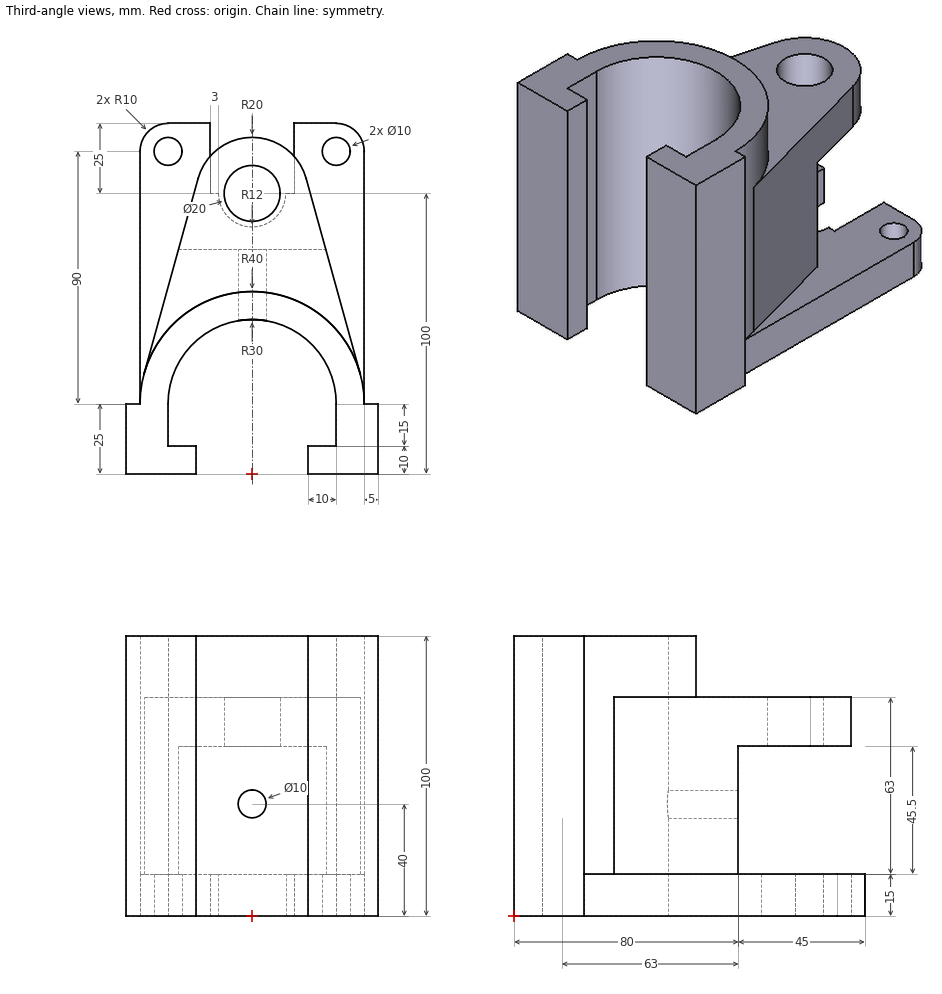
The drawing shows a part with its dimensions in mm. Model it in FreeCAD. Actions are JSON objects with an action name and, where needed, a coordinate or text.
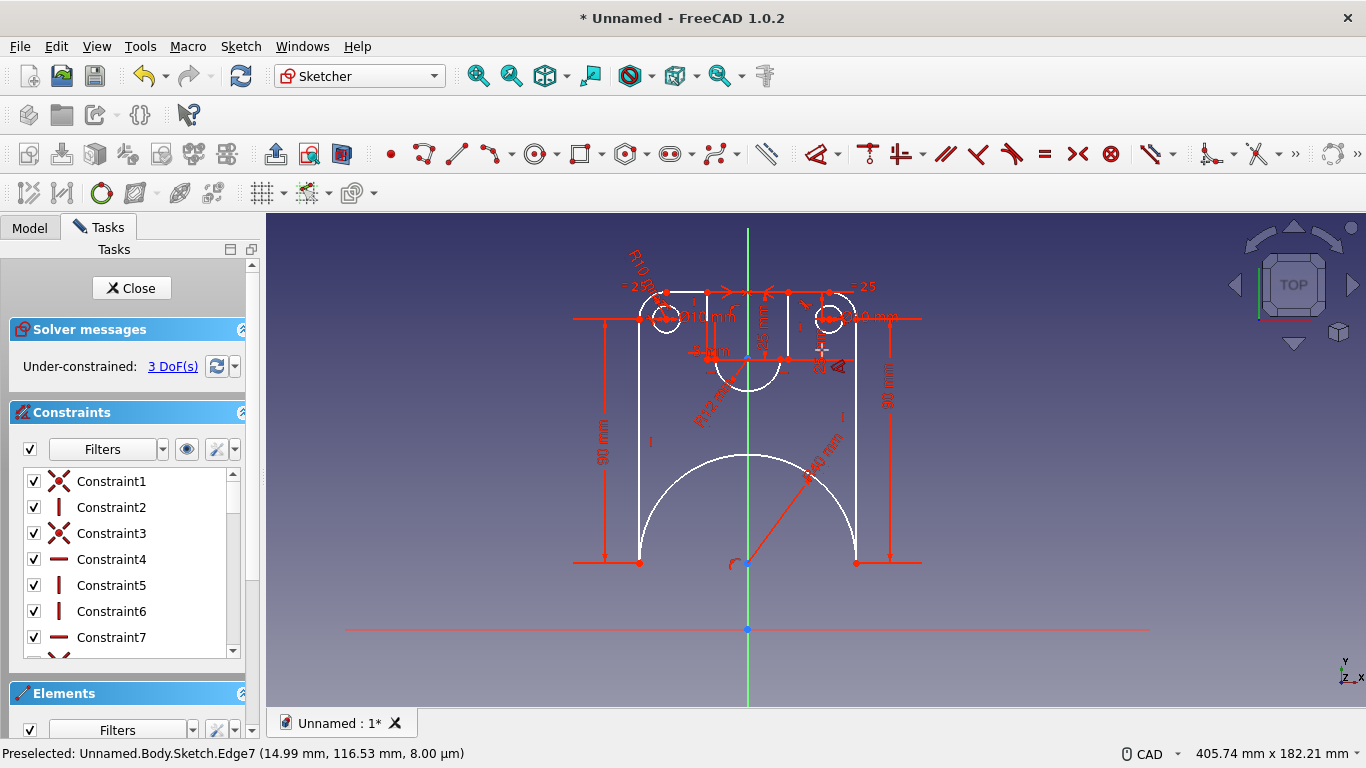
{"action": "left_click", "coordinate": [639, 563]}
{"action": "left_click", "coordinate": [605, 597]}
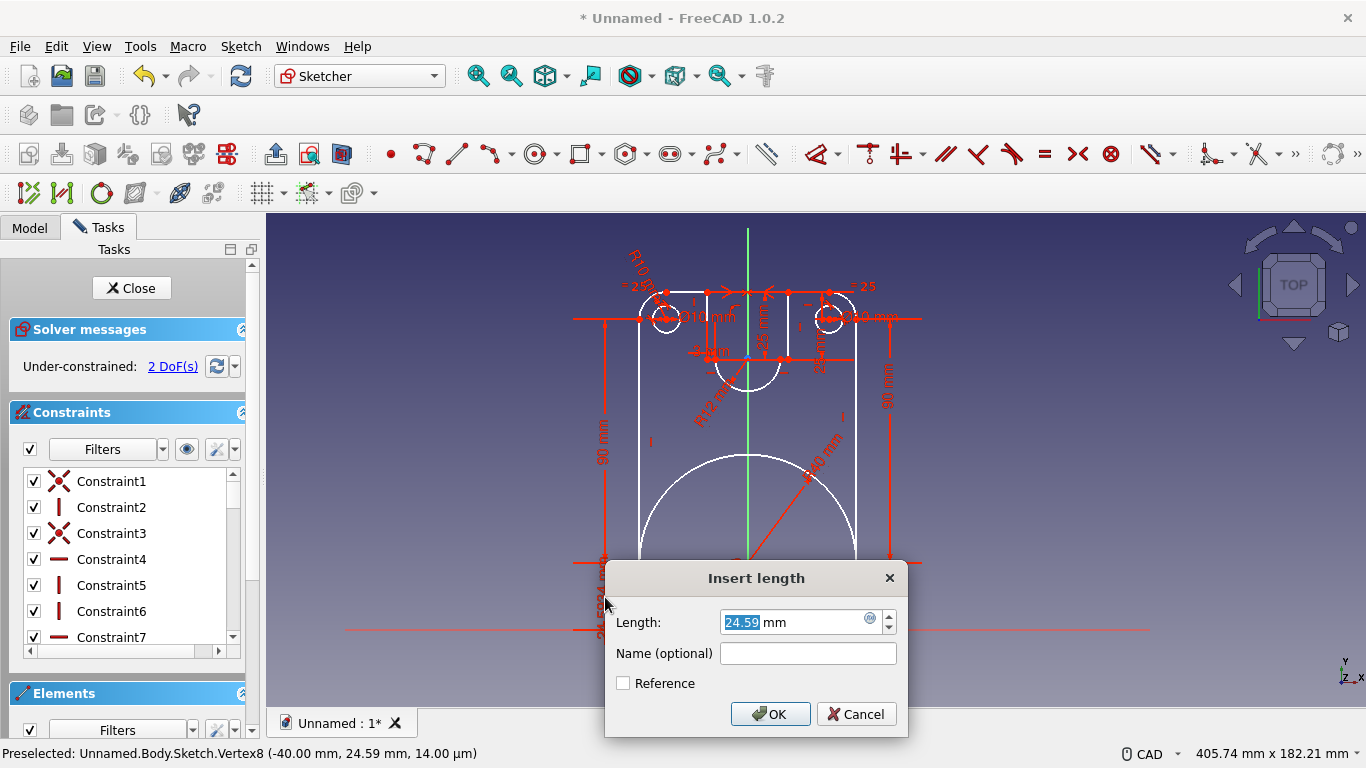
{"action": "type", "text": "25"}
{"action": "key", "text": "Return"}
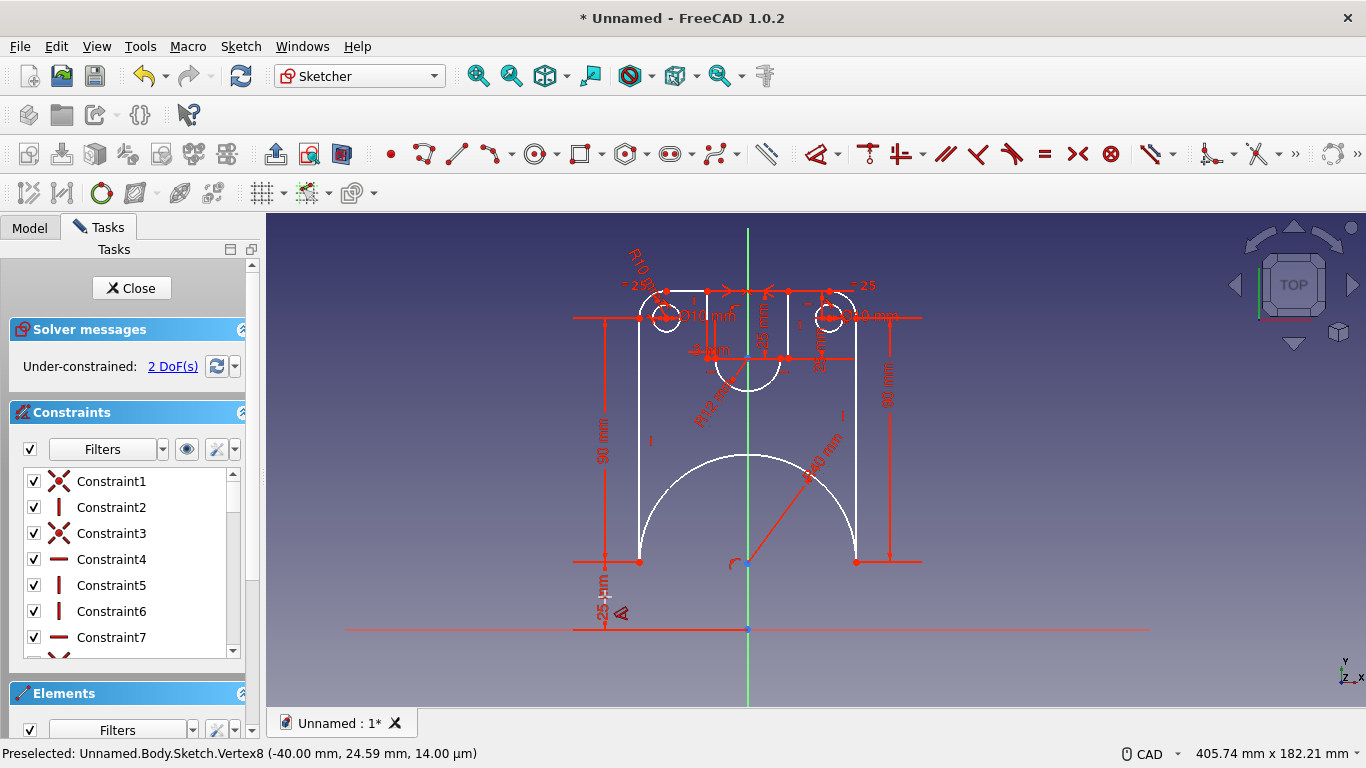
{"action": "left_click", "coordinate": [748, 563]}
{"action": "left_click", "coordinate": [782, 597]}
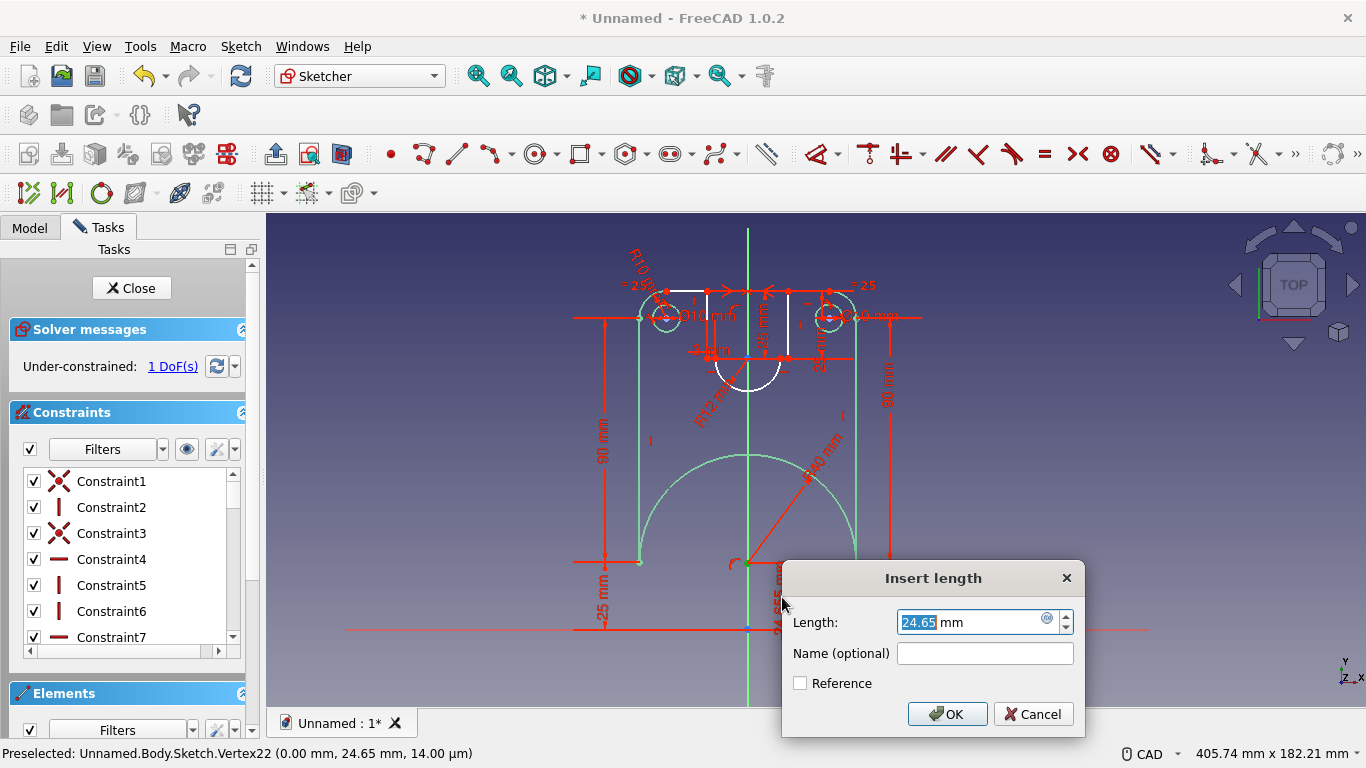
{"action": "type", "text": "25"}
{"action": "key", "text": "Return"}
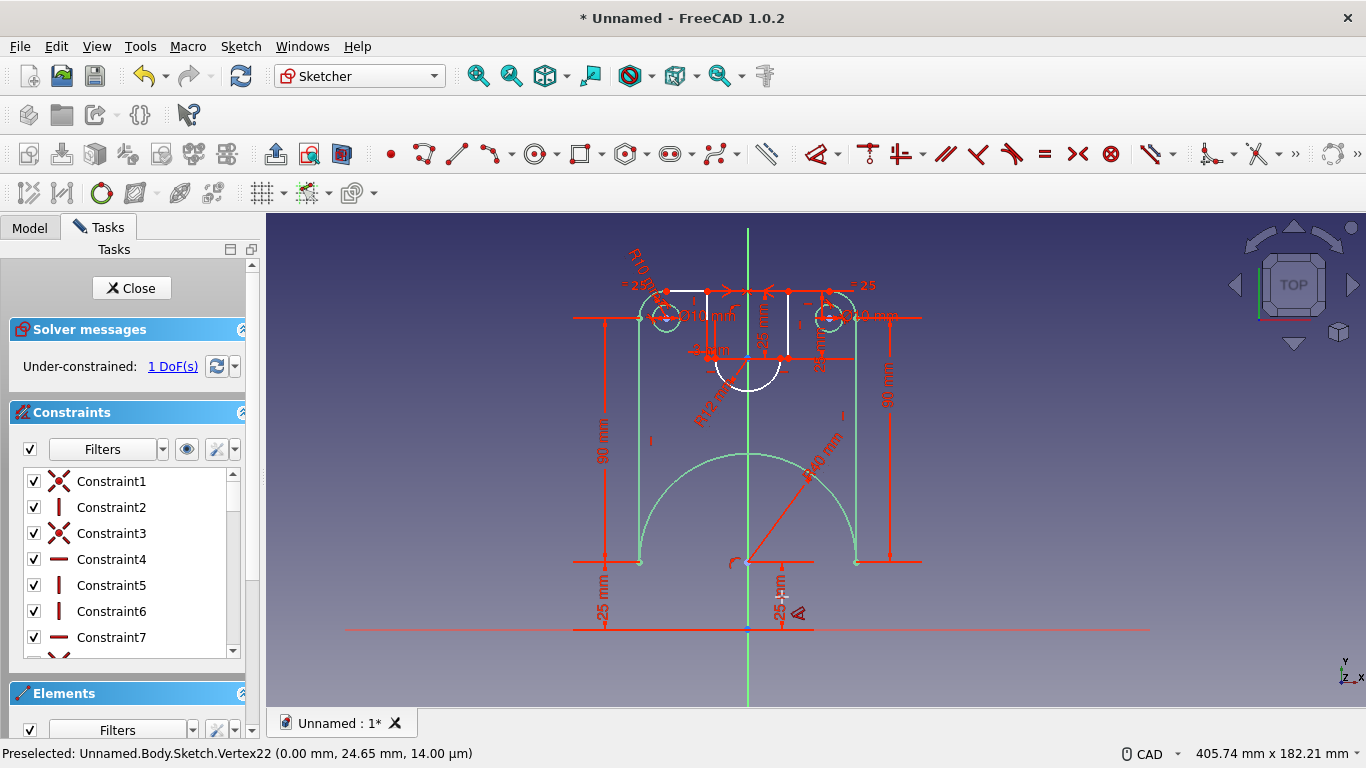
{"action": "left_click", "coordinate": [748, 359]}
{"action": "left_click", "coordinate": [782, 494]}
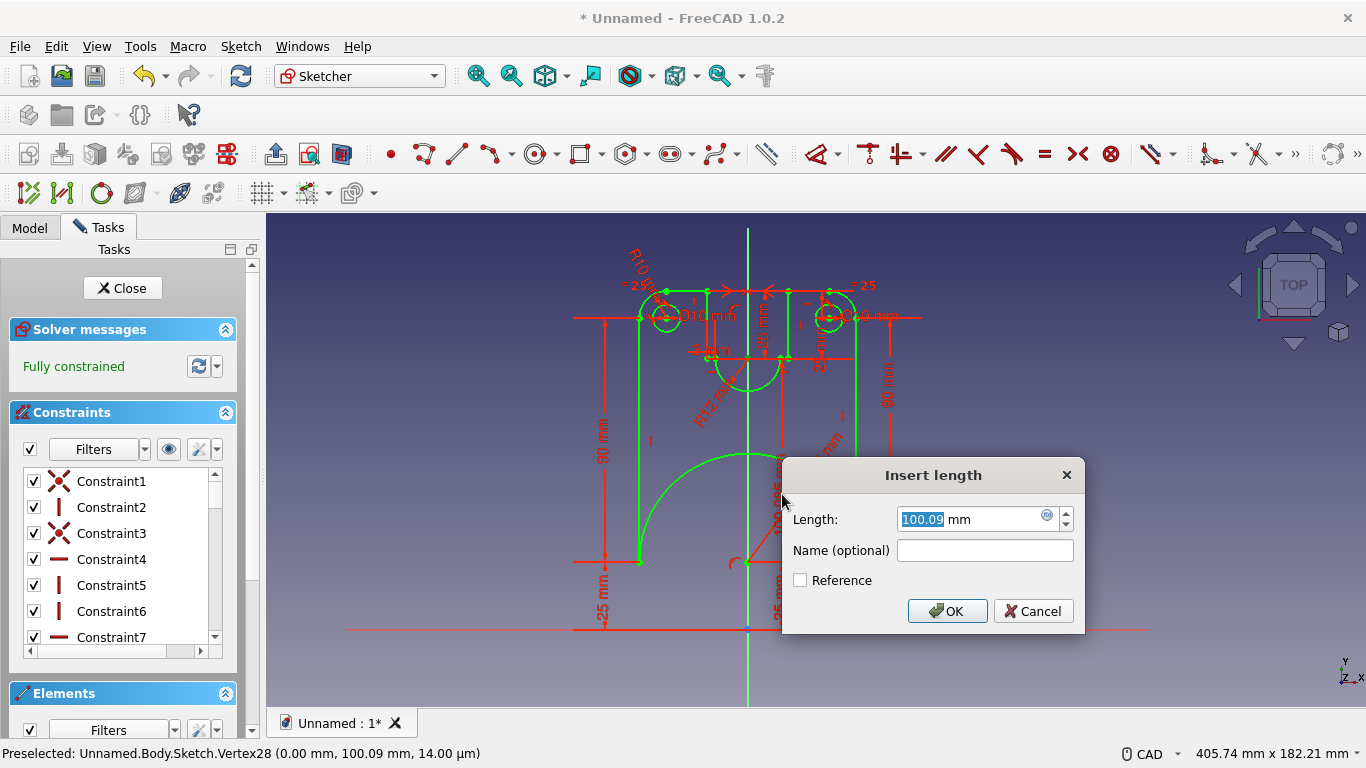
{"action": "type", "text": "100"}
{"action": "key", "text": "Return"}
{"action": "key", "text": "Escape"}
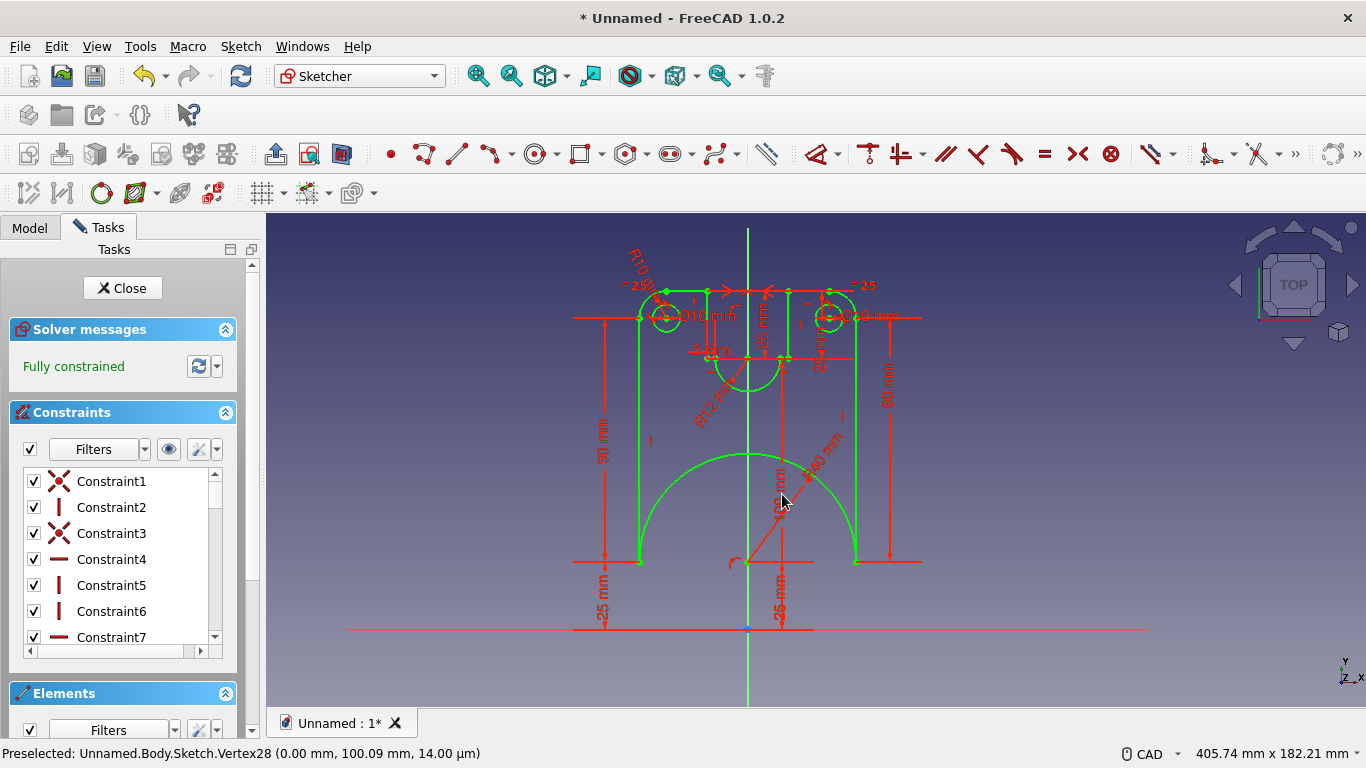
{"action": "left_click", "coordinate": [123, 288]}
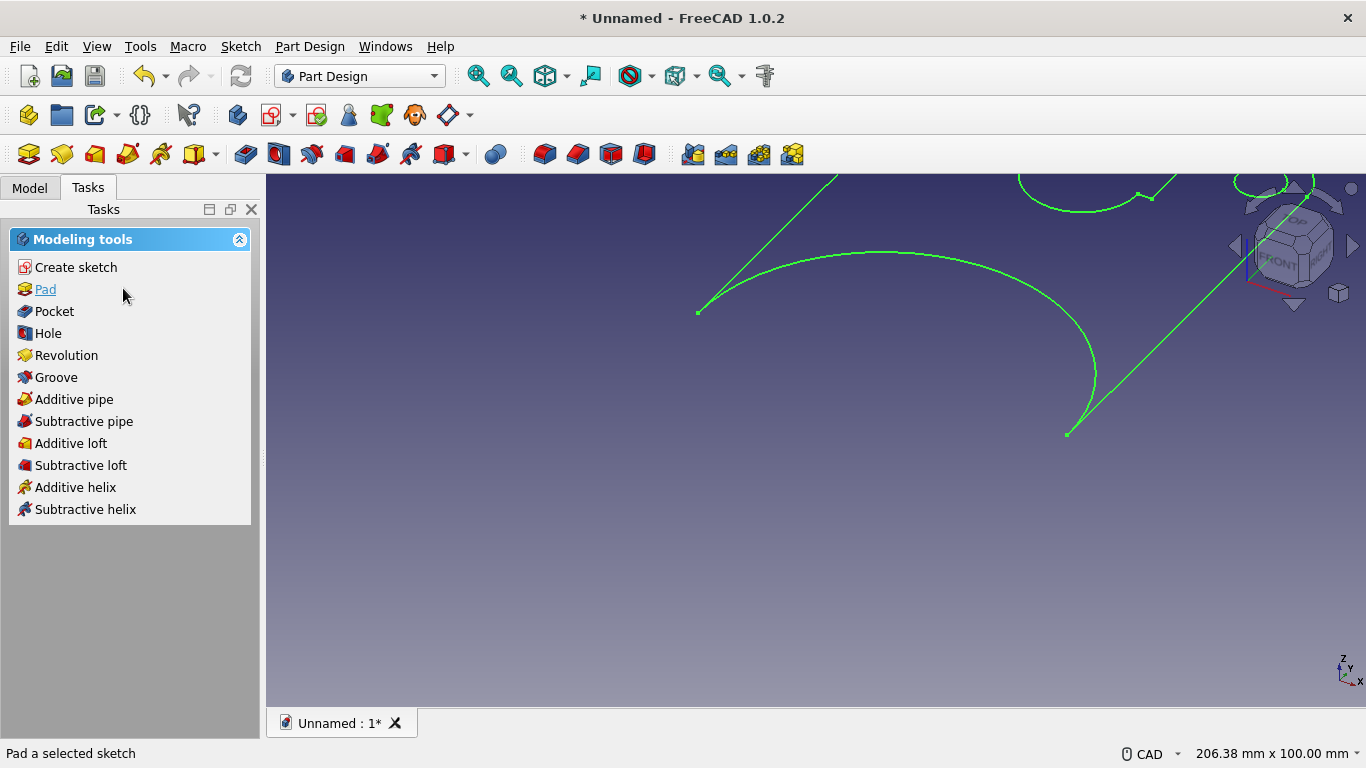
{"action": "left_click", "coordinate": [29, 154]}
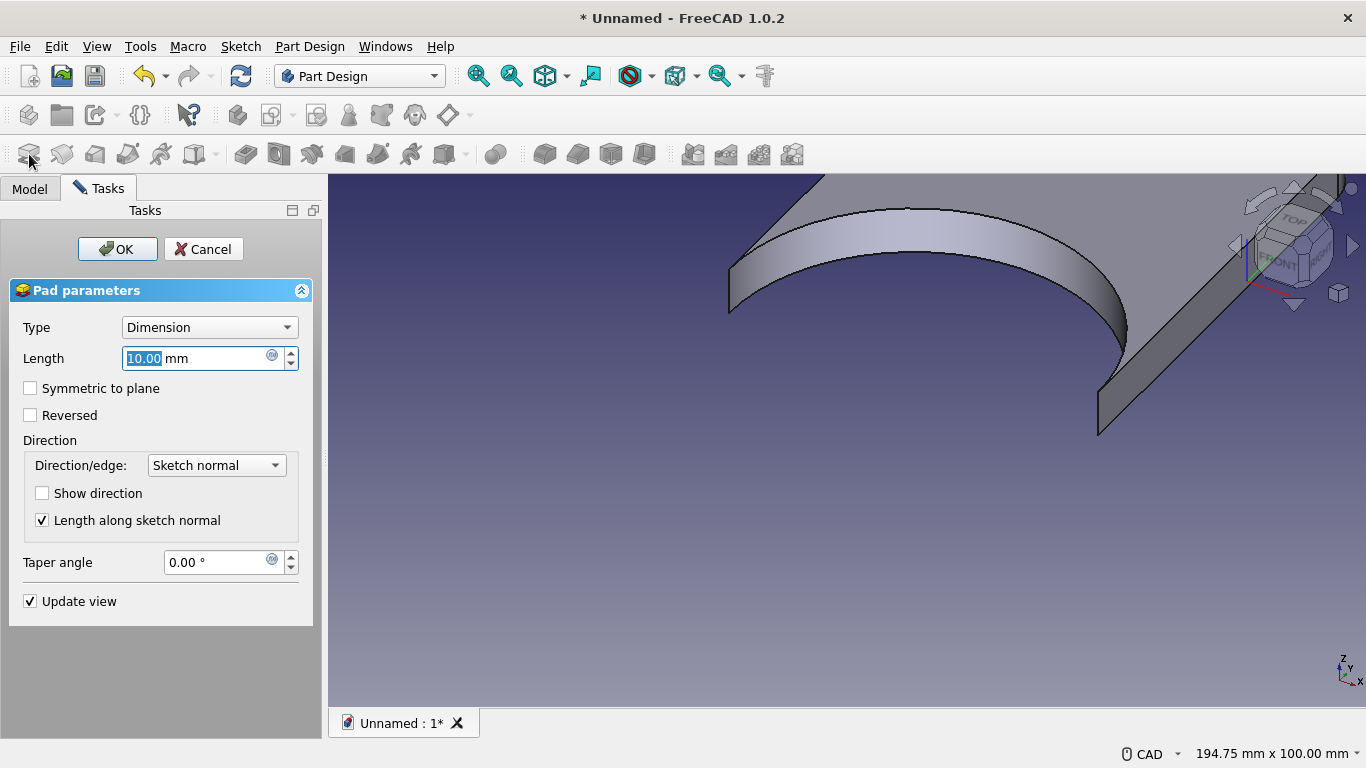
{"action": "type", "text": "15"}
{"action": "key", "text": "Tab"}